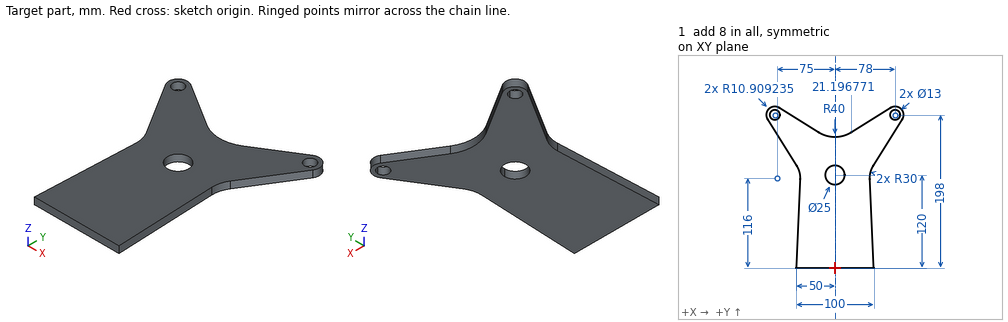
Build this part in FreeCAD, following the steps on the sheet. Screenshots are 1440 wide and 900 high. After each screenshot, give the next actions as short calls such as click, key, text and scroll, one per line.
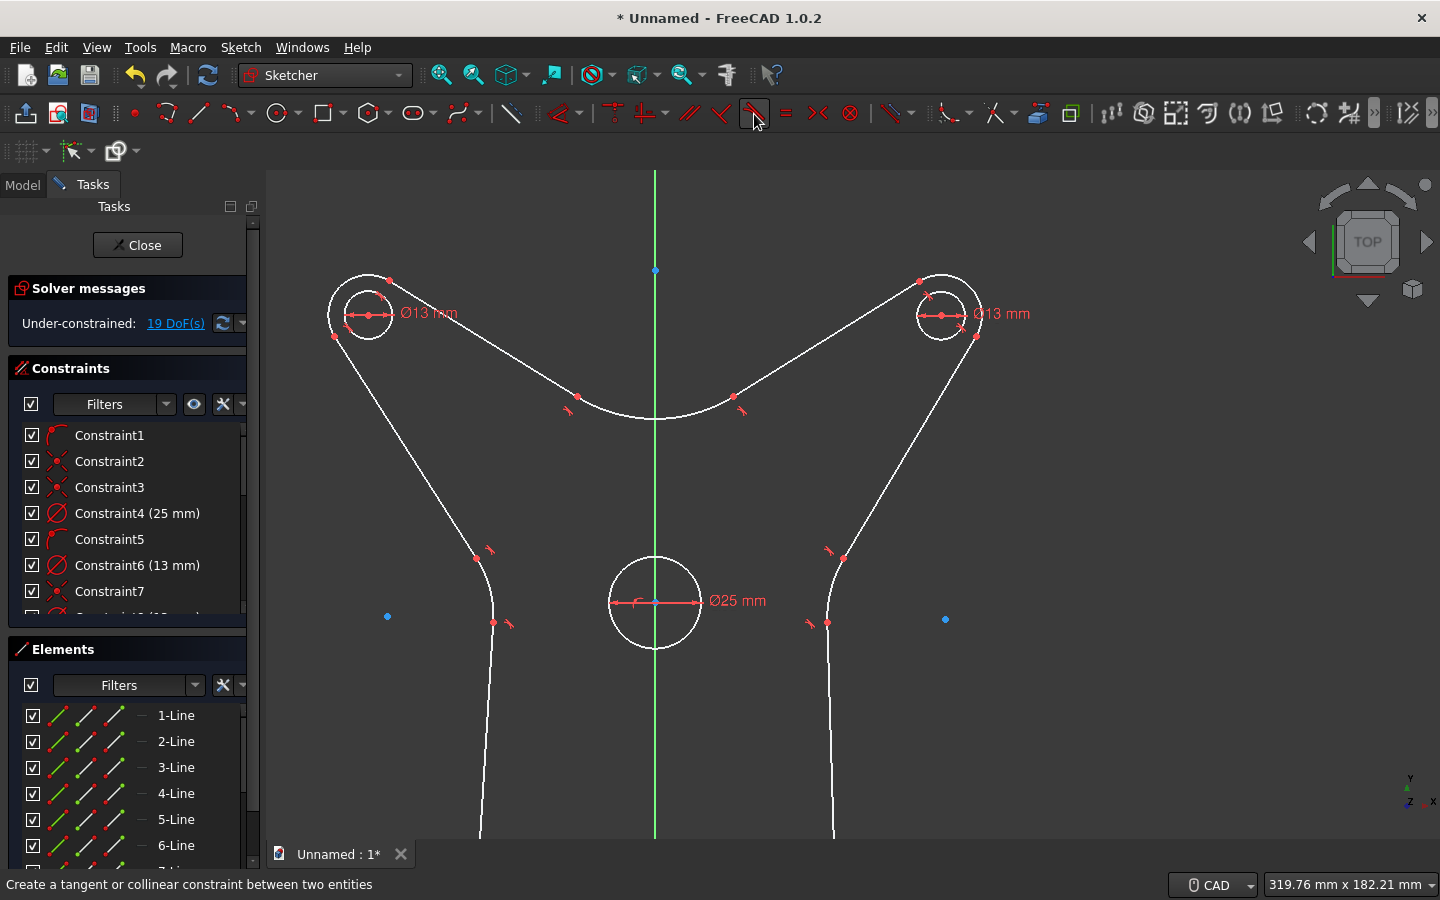
scroll(942, 314, down, 3)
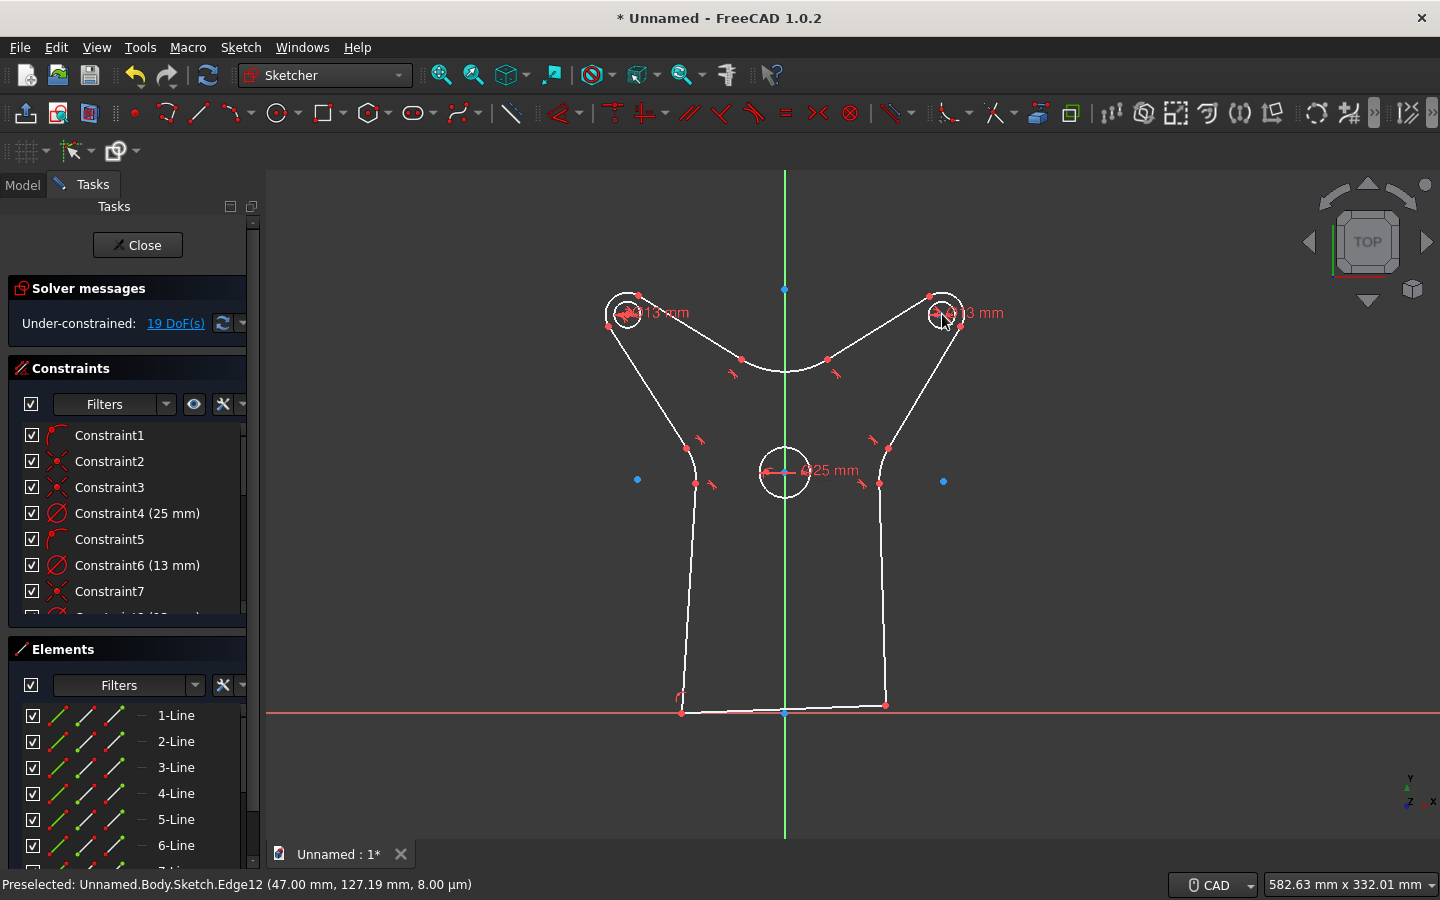
scroll(825, 708, up, 5)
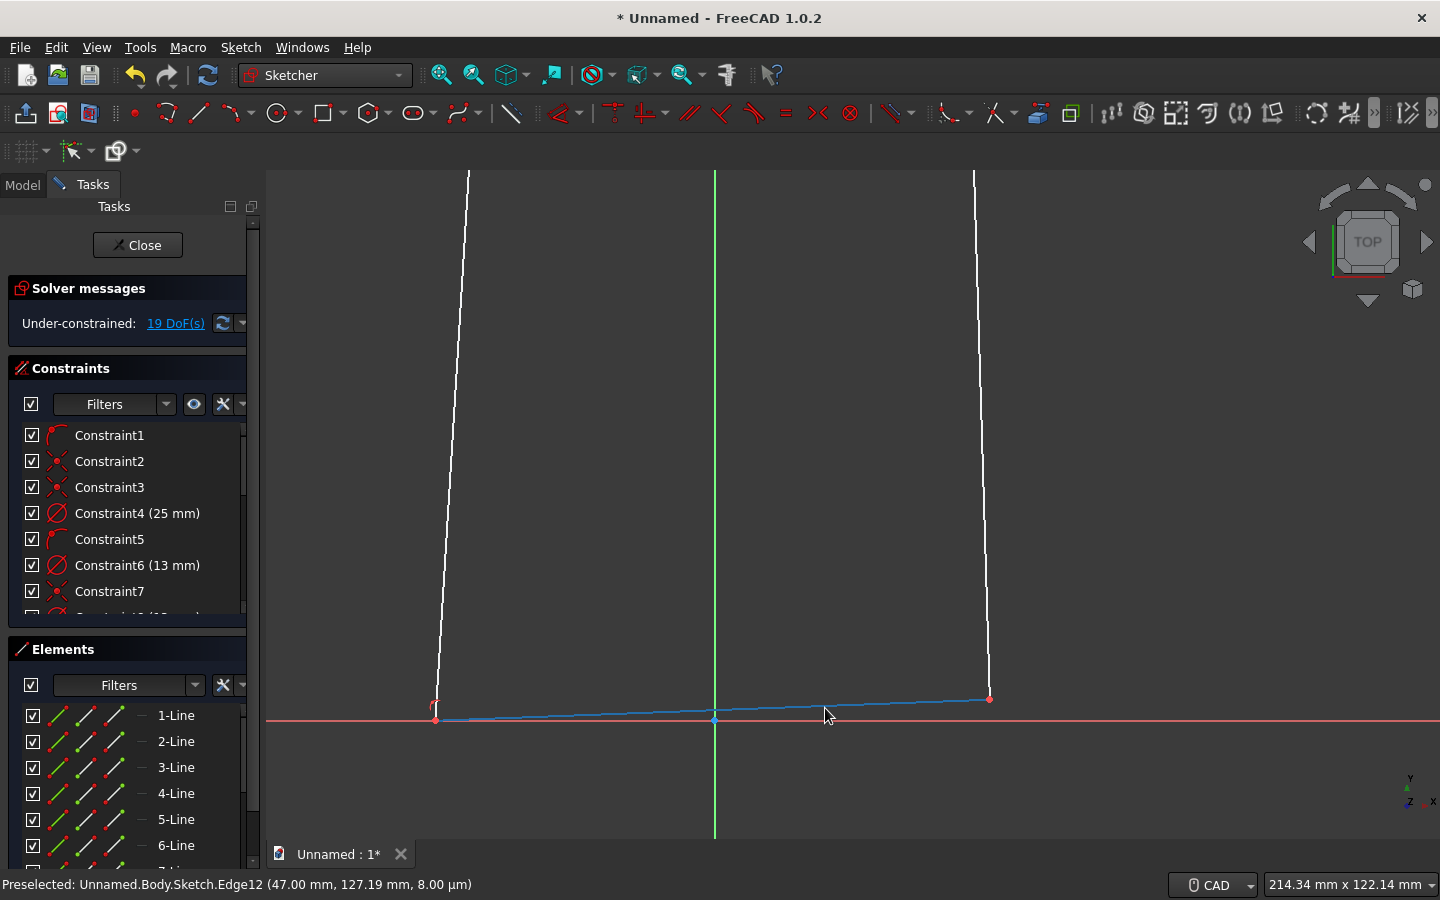
click(824, 706)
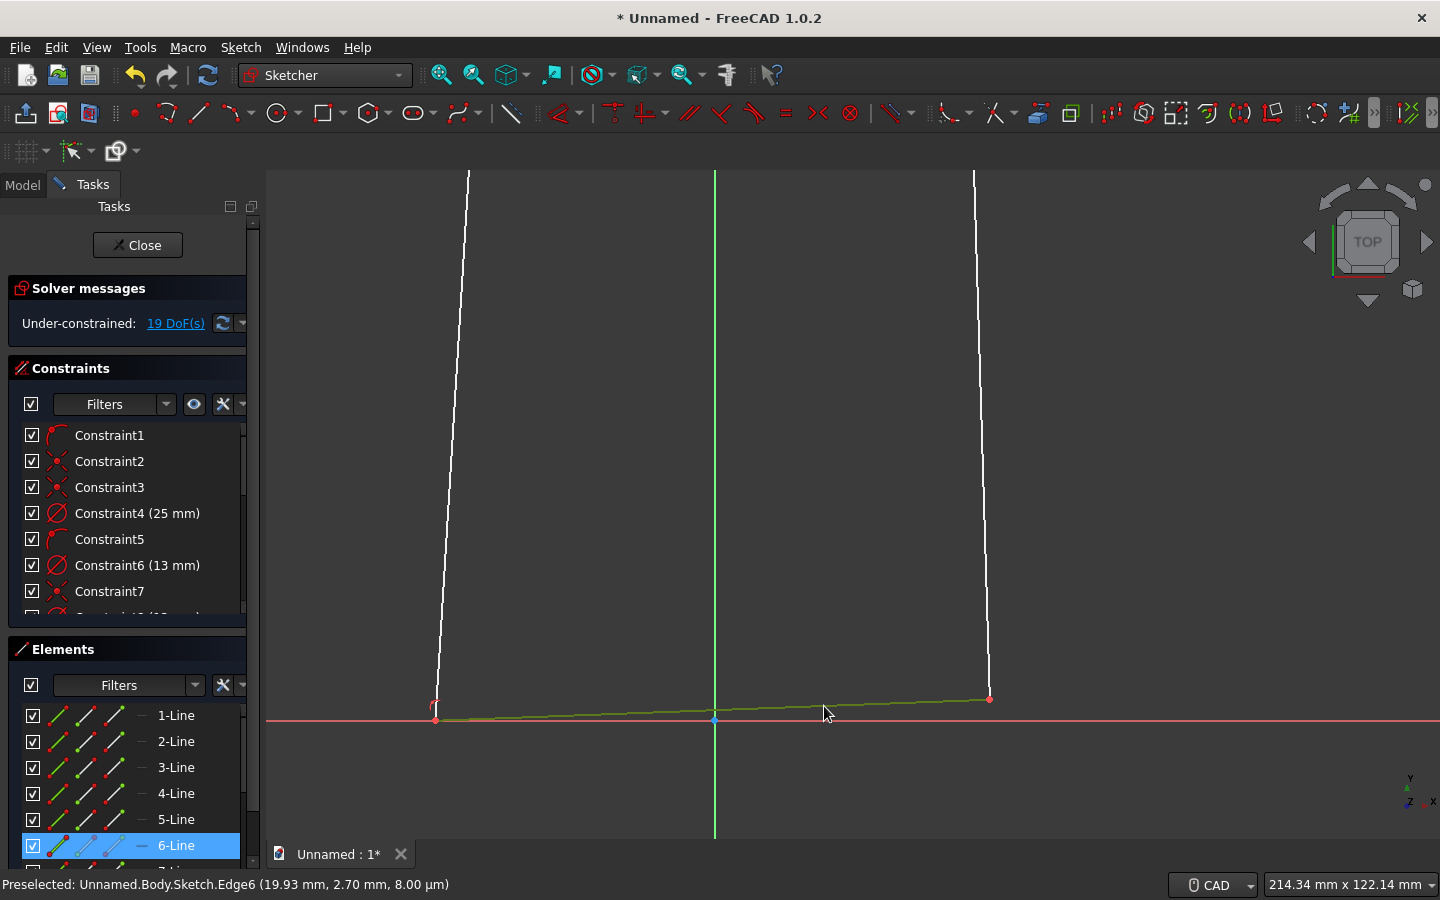
key(h)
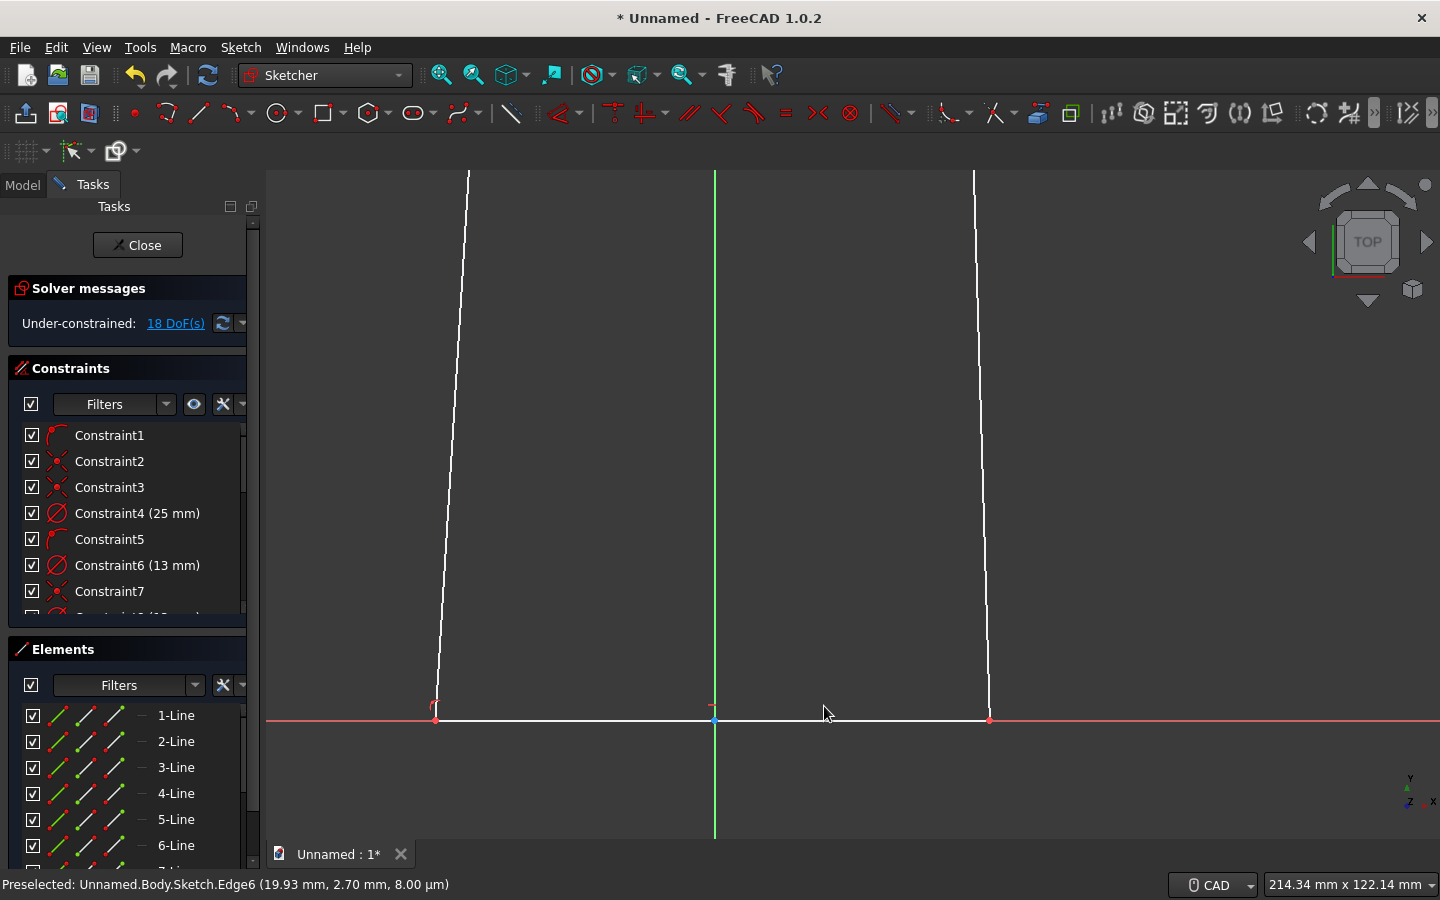
scroll(825, 709, down, 5)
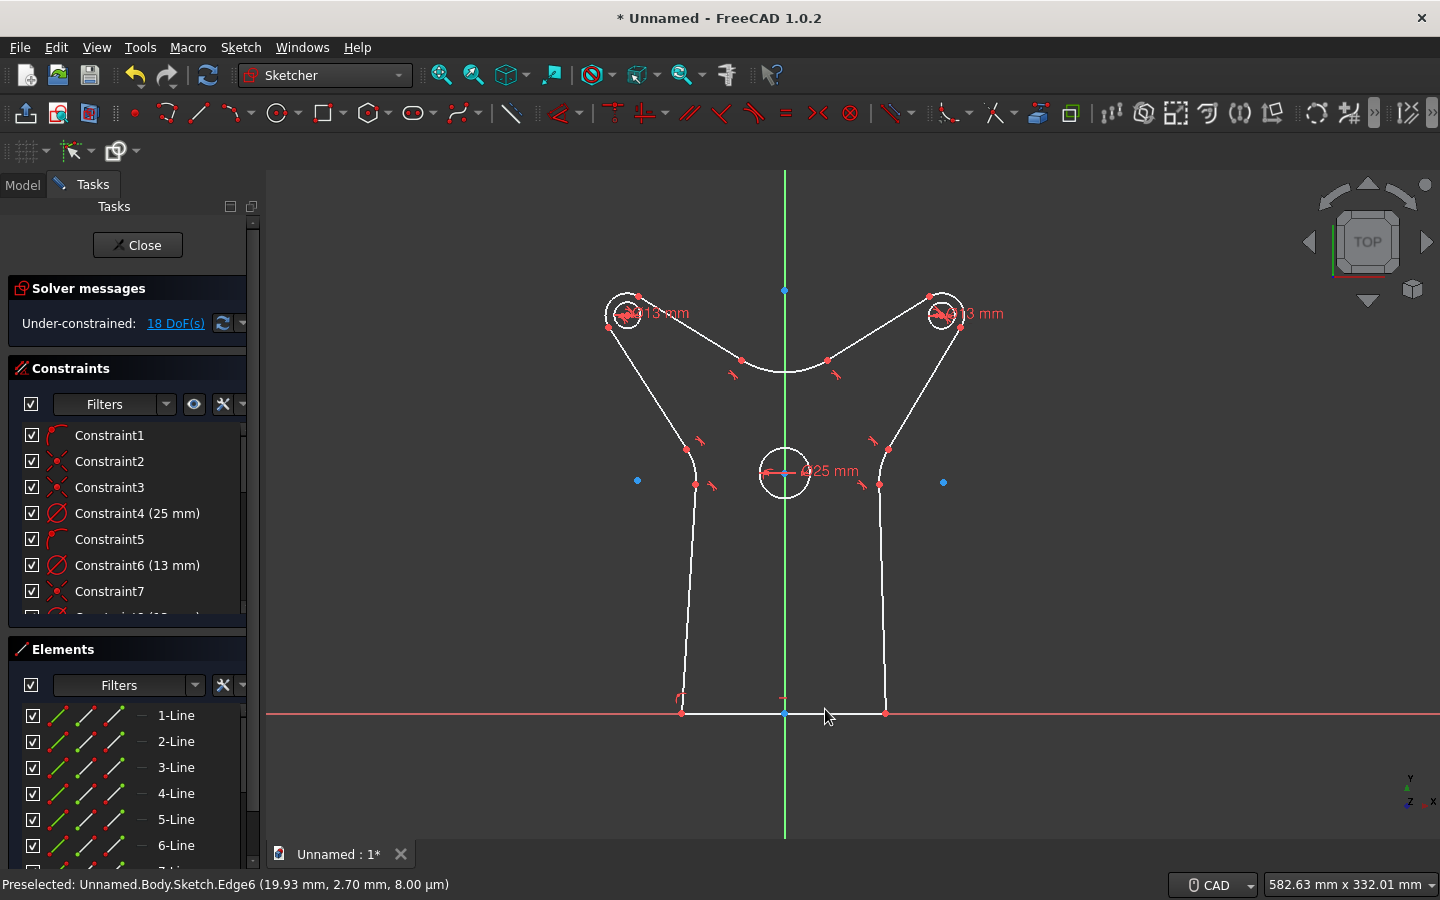
scroll(963, 310, up, 2)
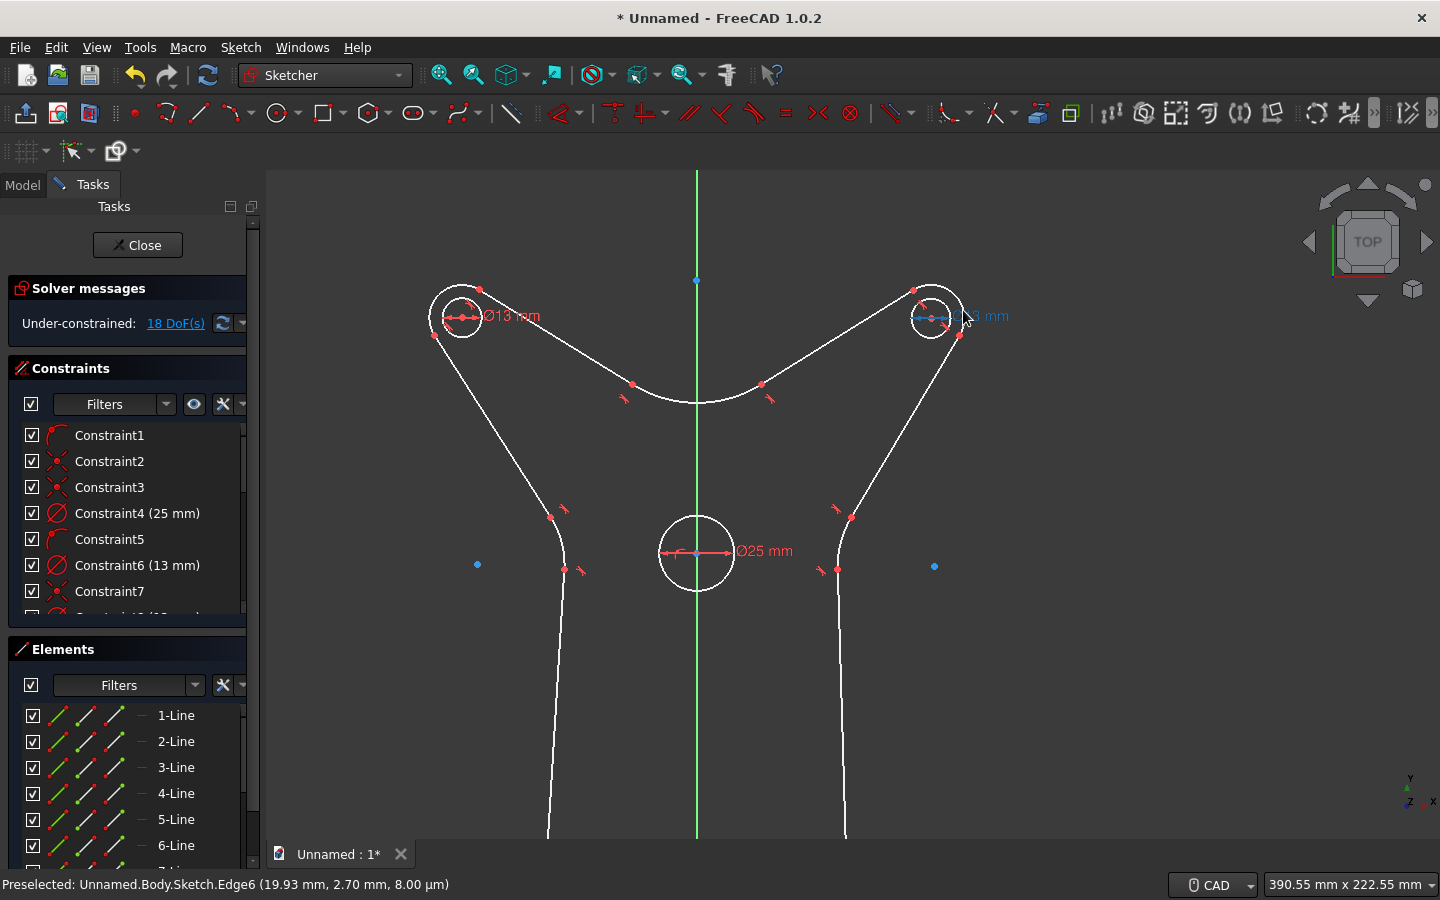
click(963, 310)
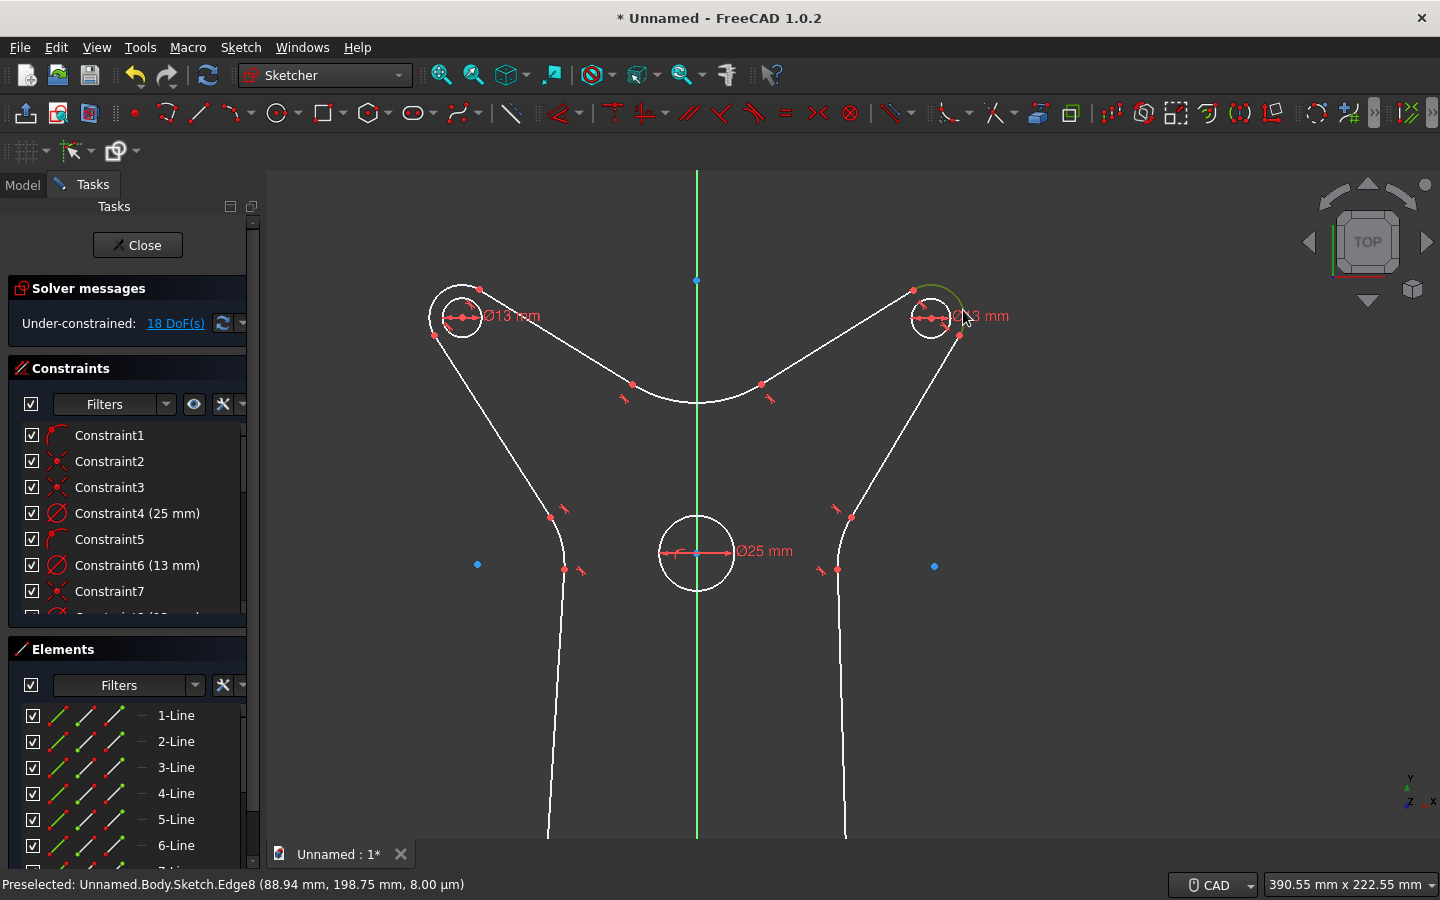
click(454, 286)